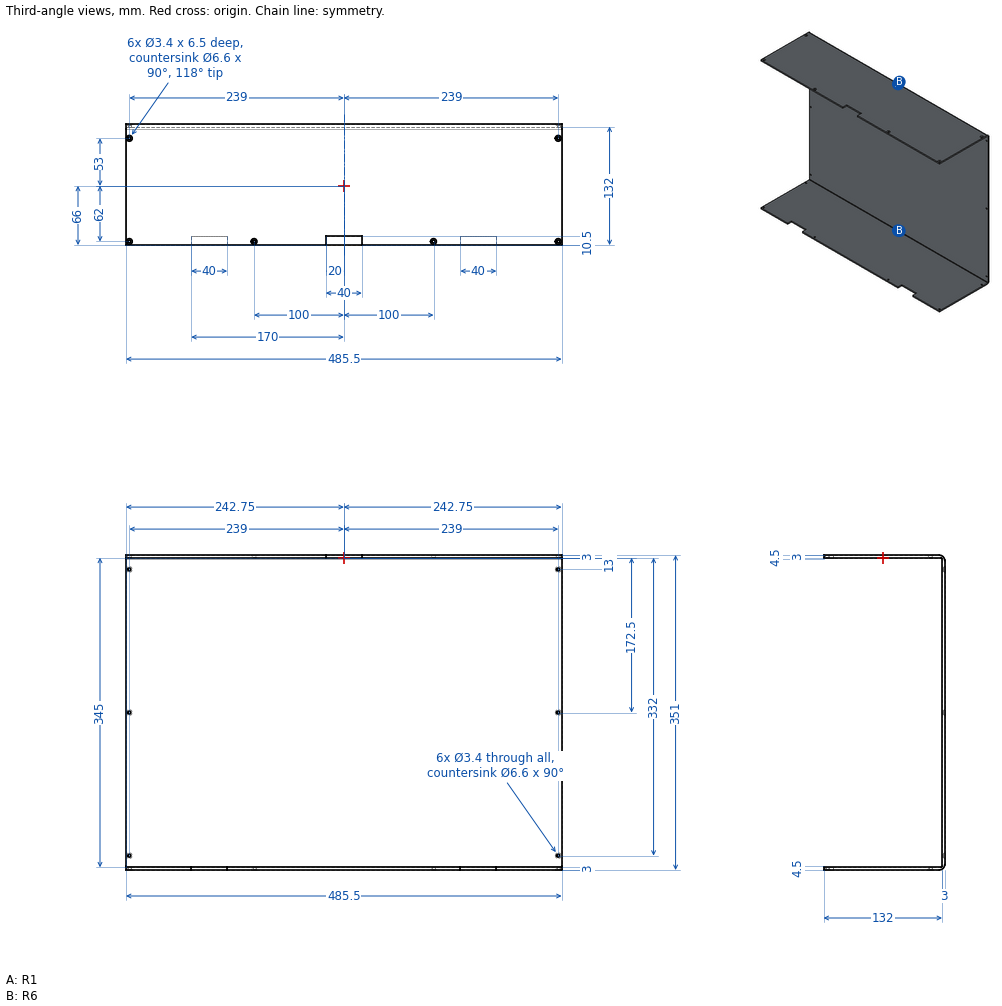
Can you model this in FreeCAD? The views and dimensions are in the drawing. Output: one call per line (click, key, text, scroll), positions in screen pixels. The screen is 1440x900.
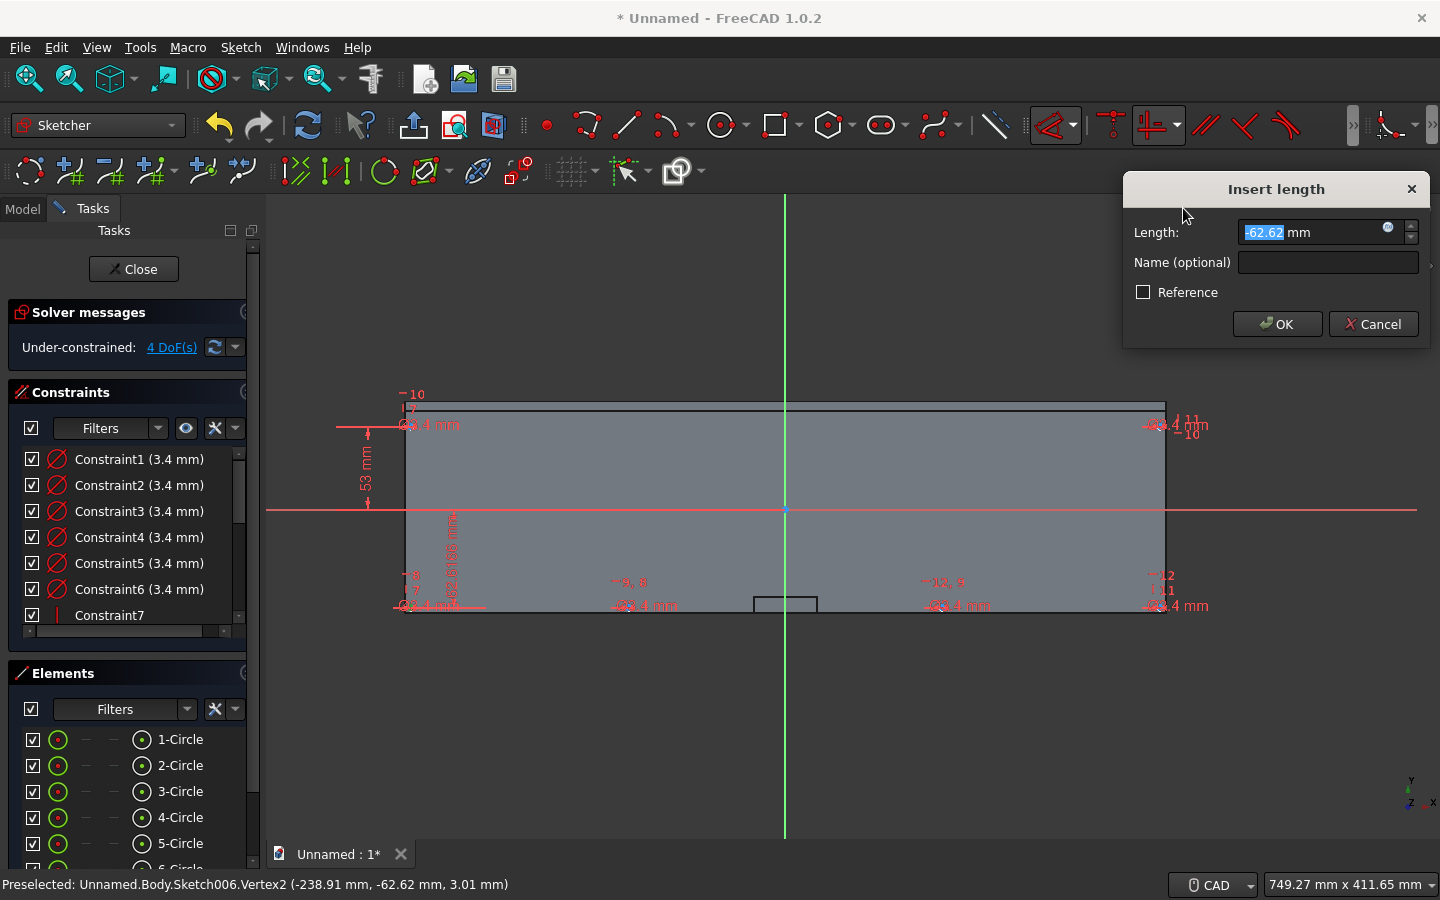
text(-62)
key(Return)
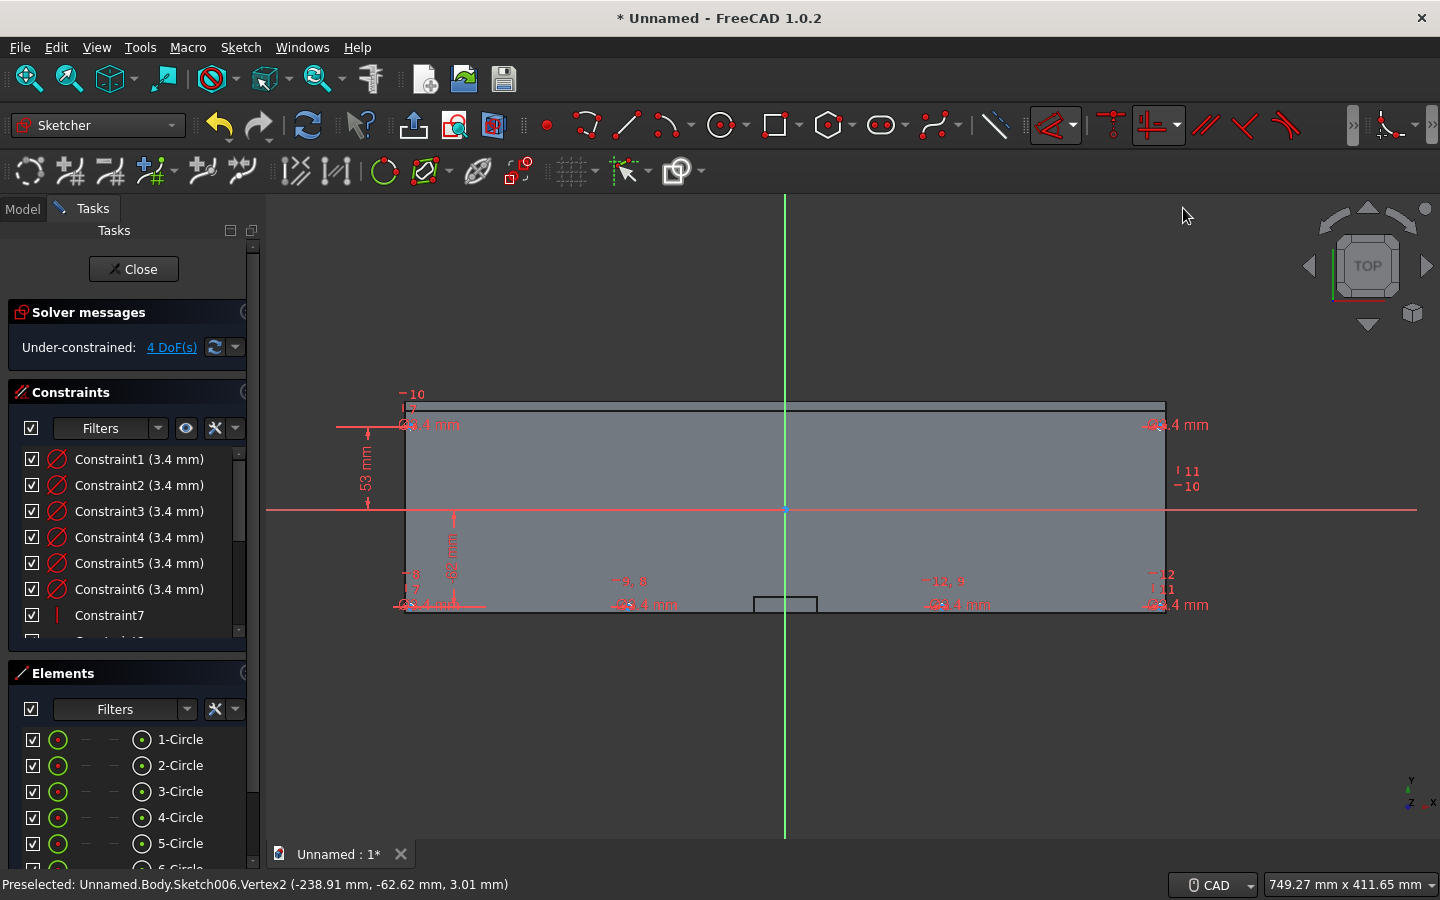
click(411, 427)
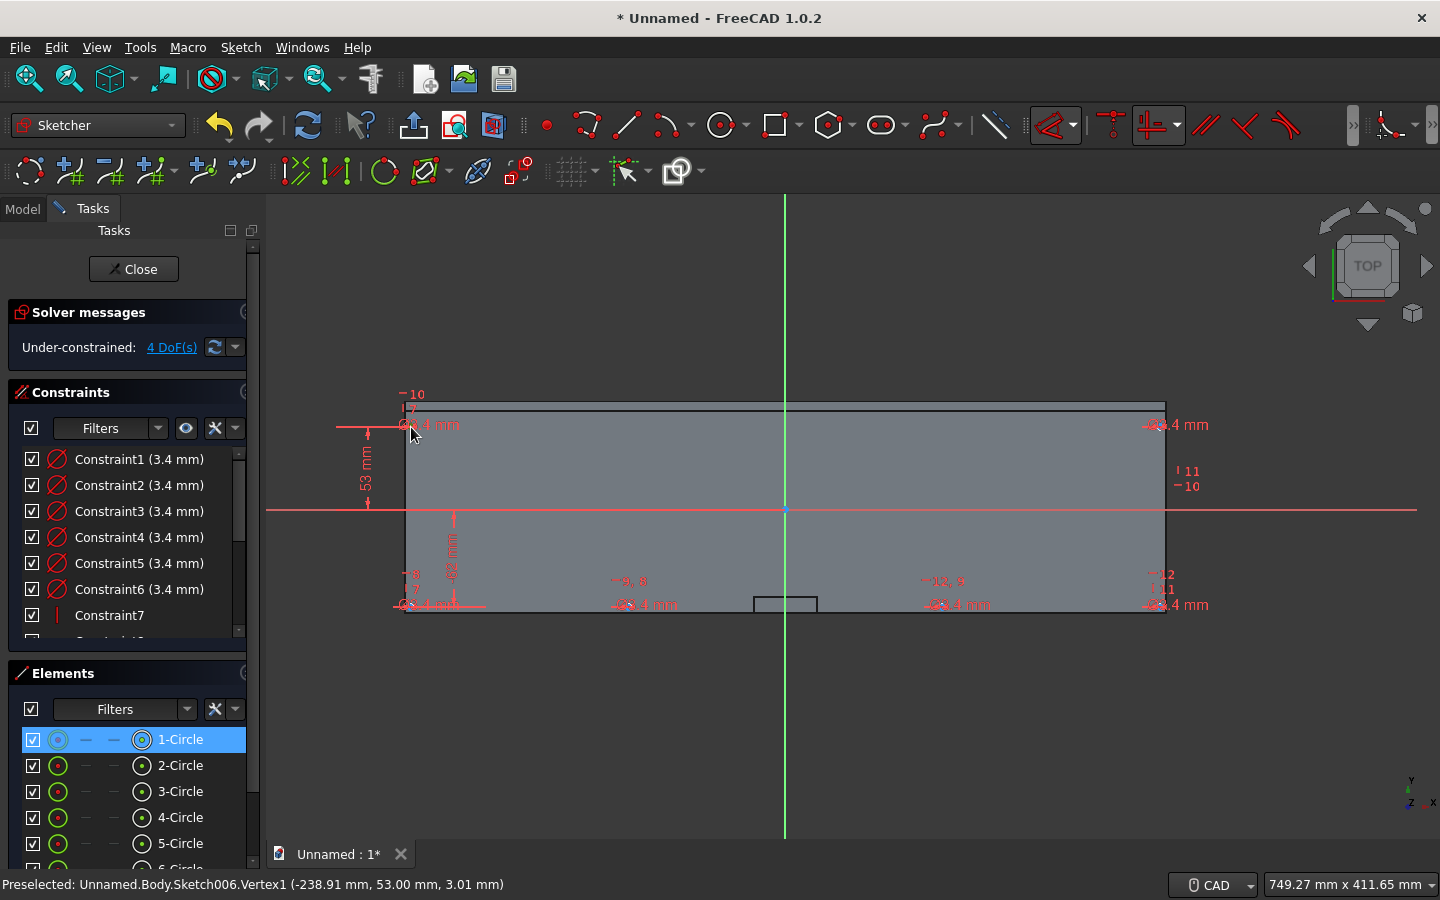
click(1076, 126)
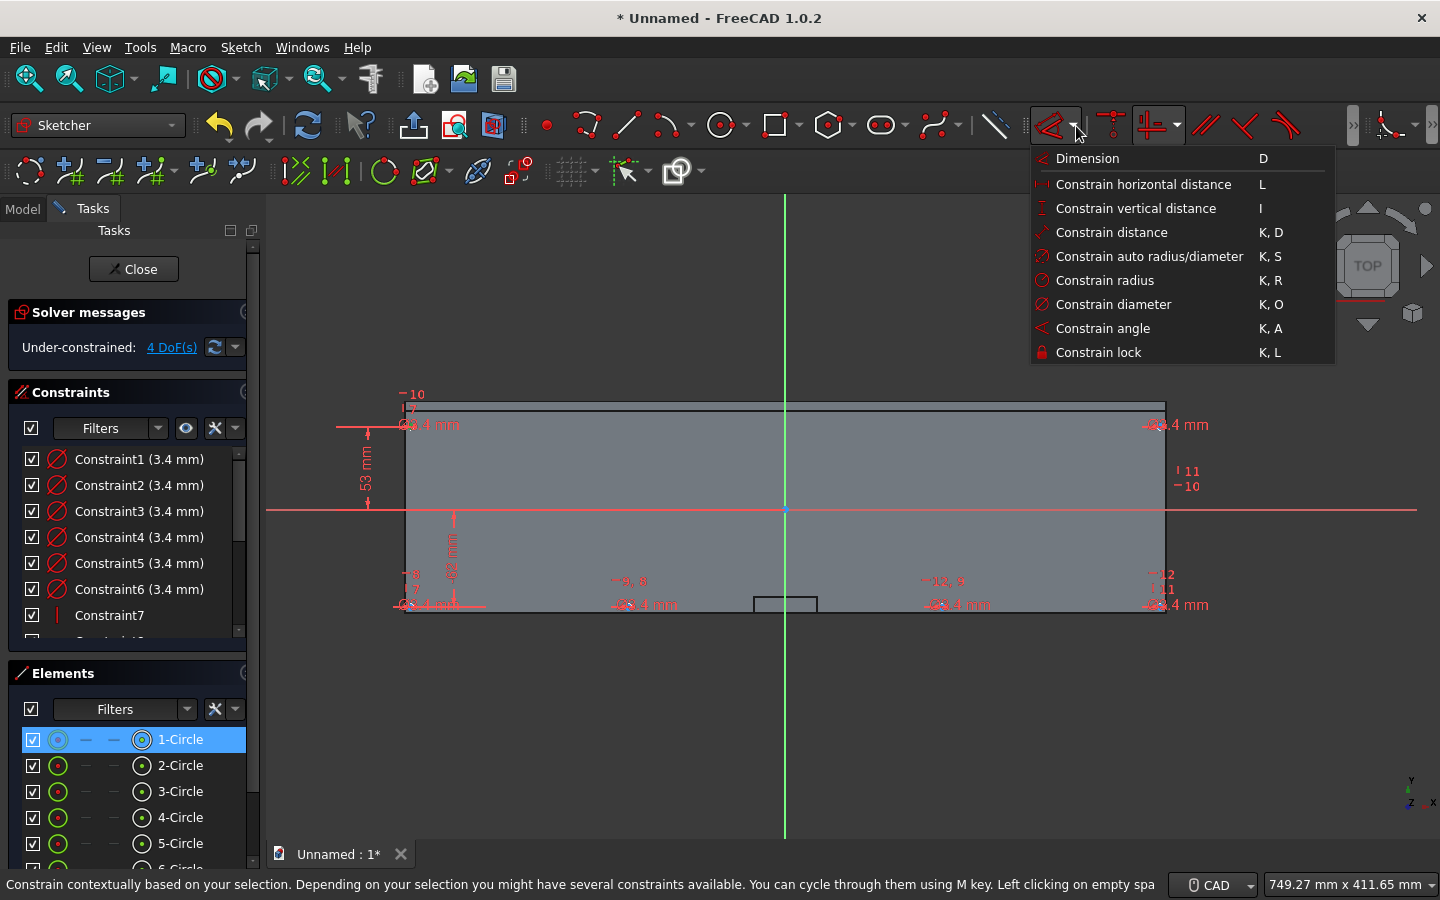
click(1183, 184)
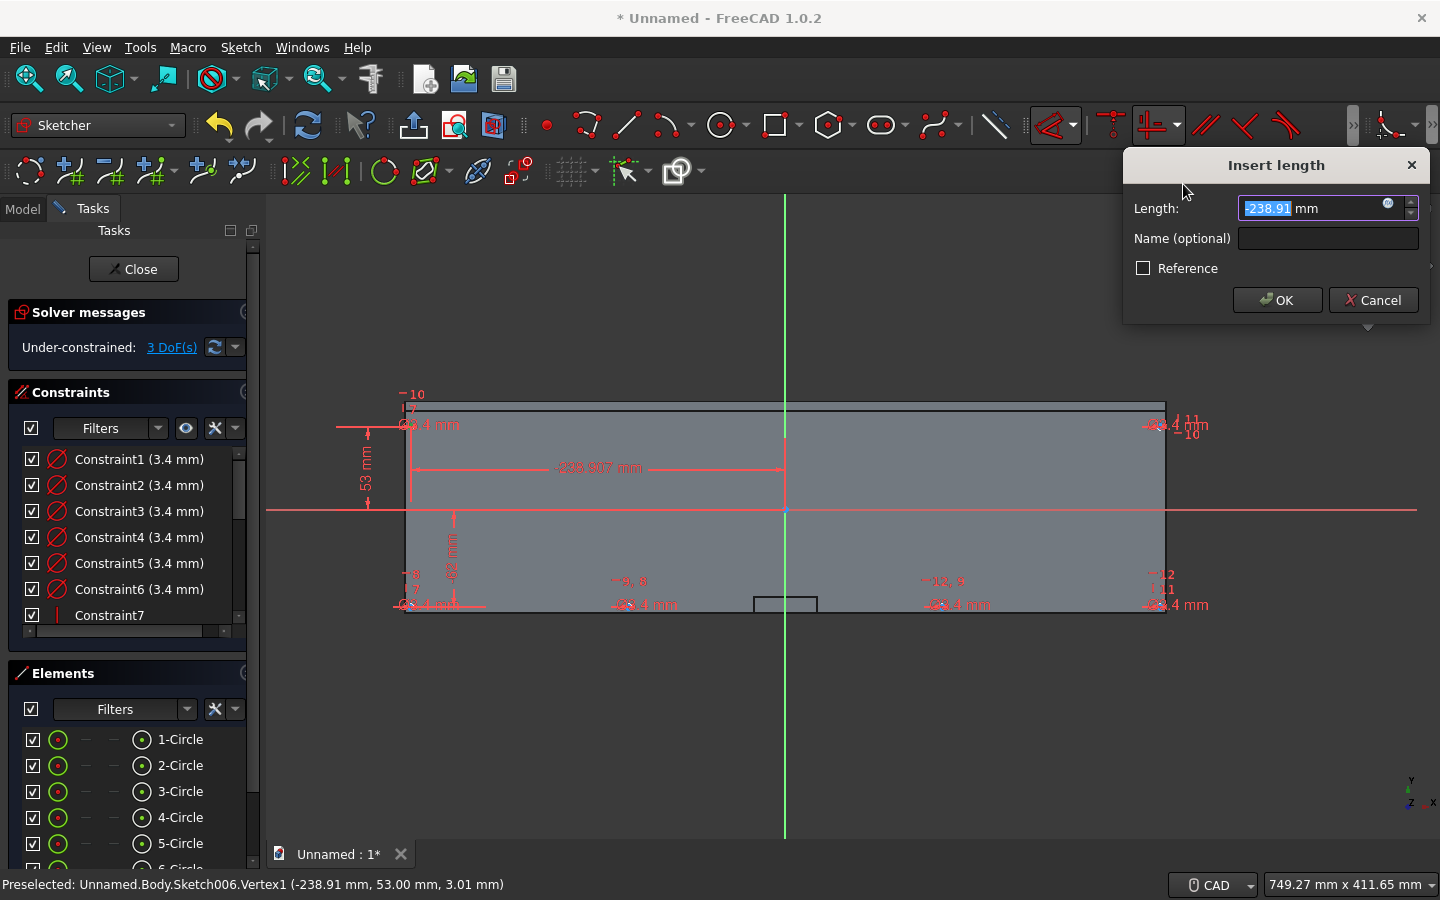
text(-239)
key(Return)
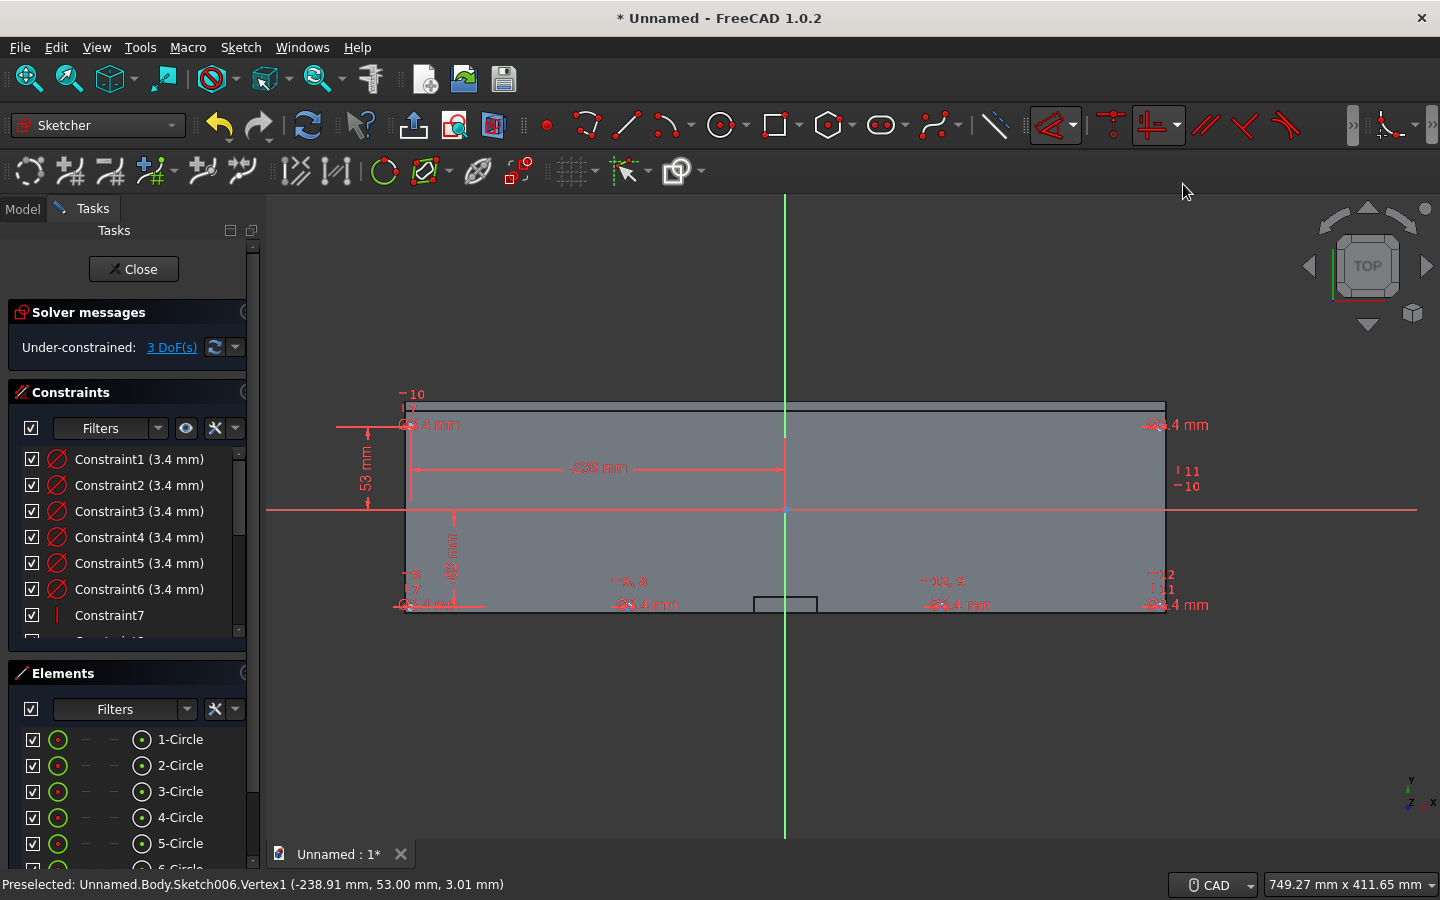
click(629, 607)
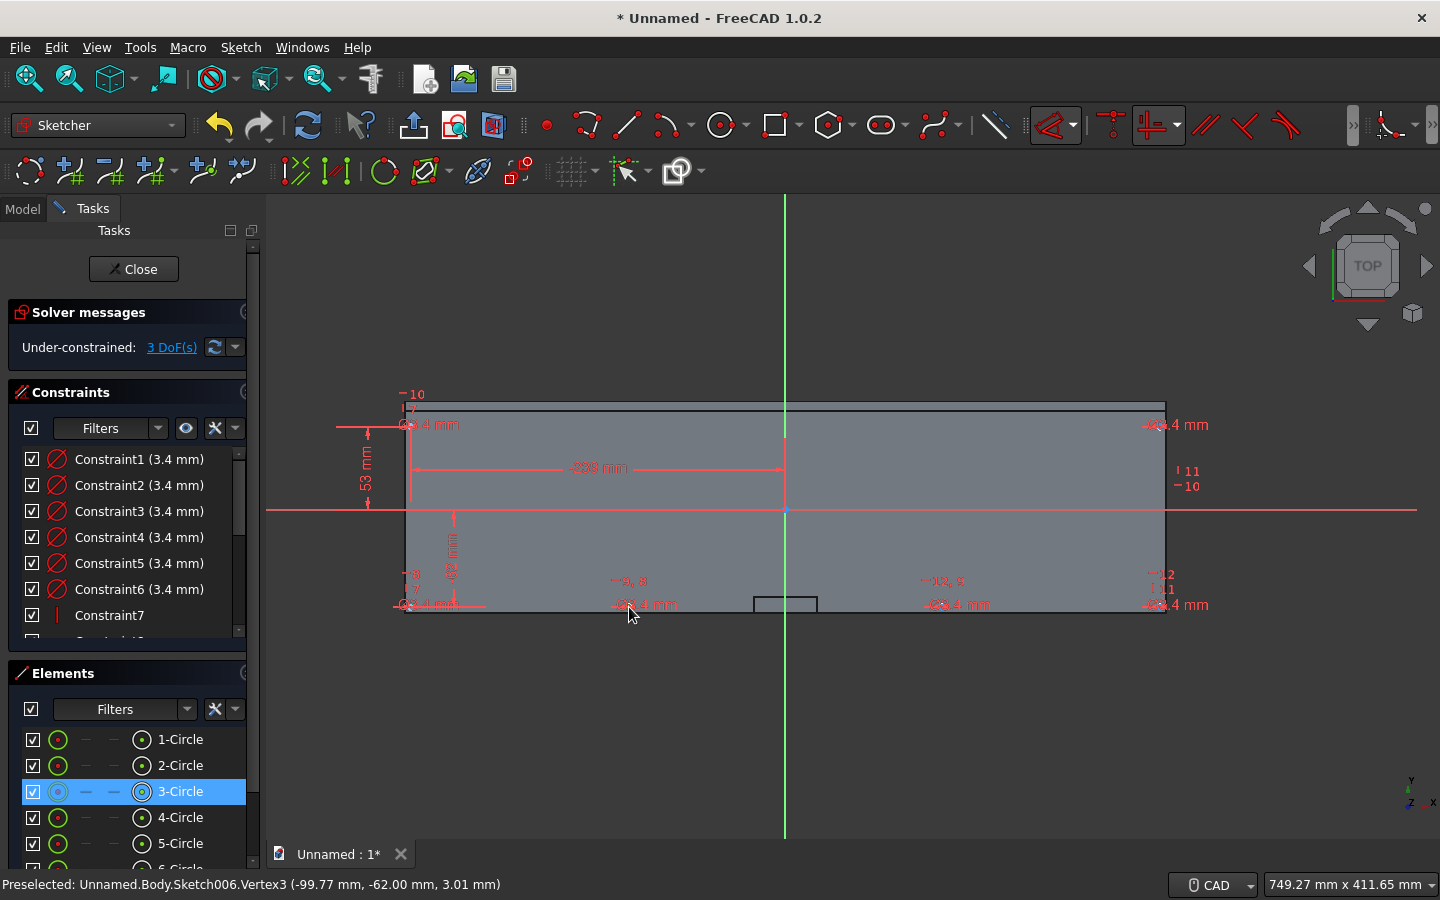
key(l)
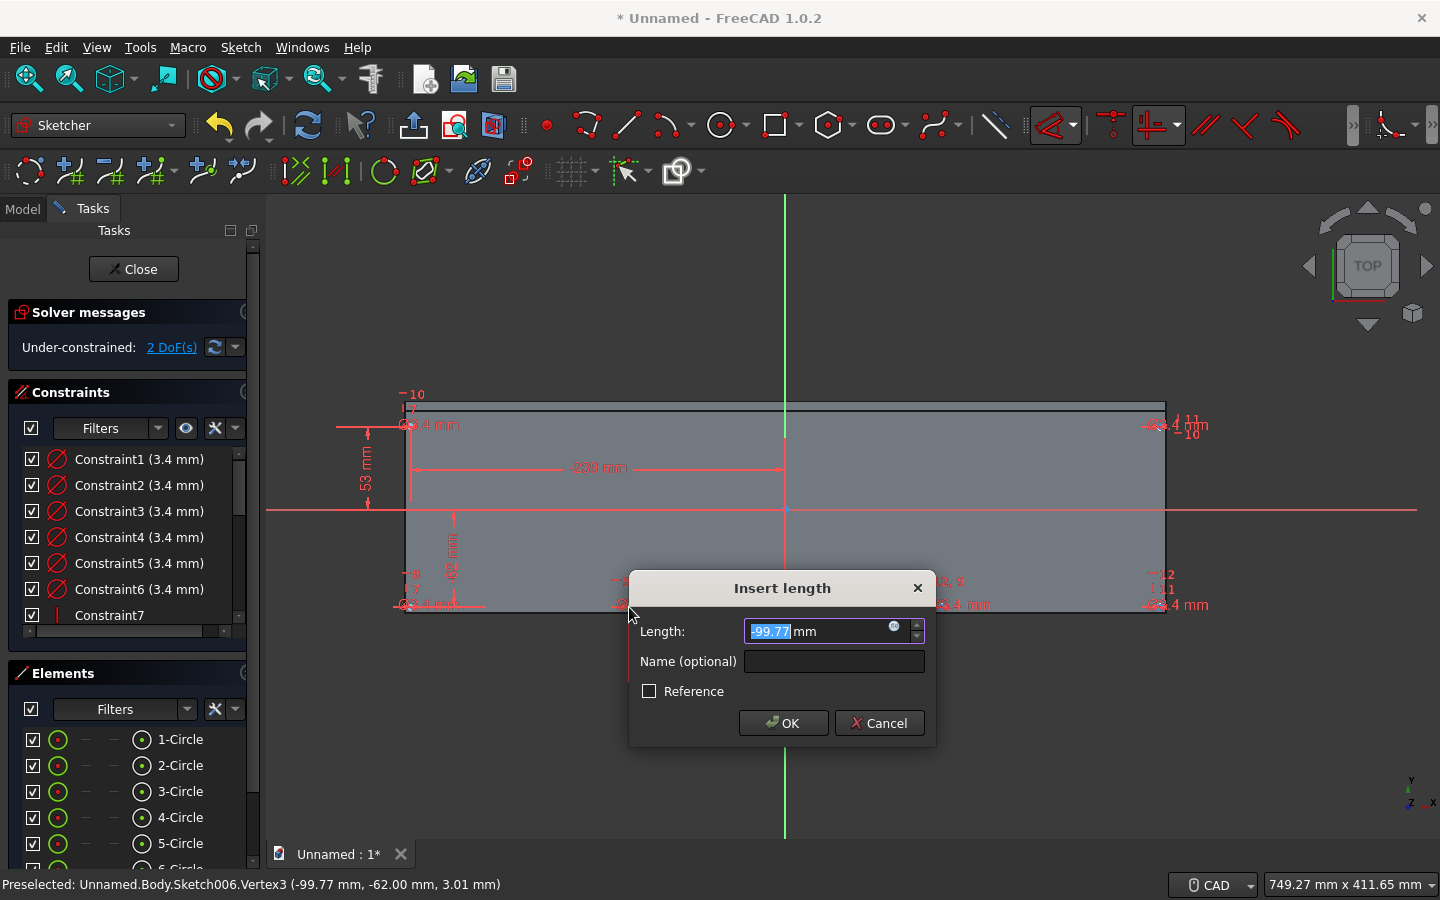
text(-100)
key(Return)